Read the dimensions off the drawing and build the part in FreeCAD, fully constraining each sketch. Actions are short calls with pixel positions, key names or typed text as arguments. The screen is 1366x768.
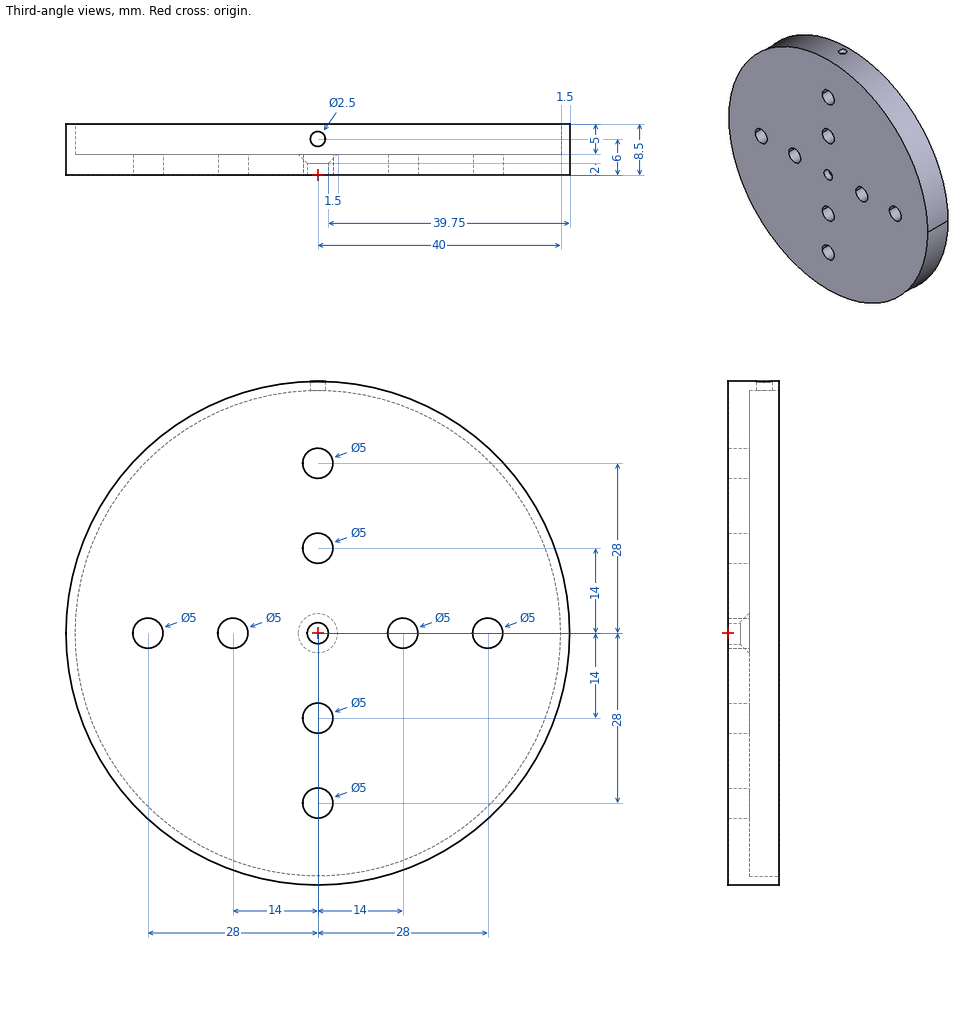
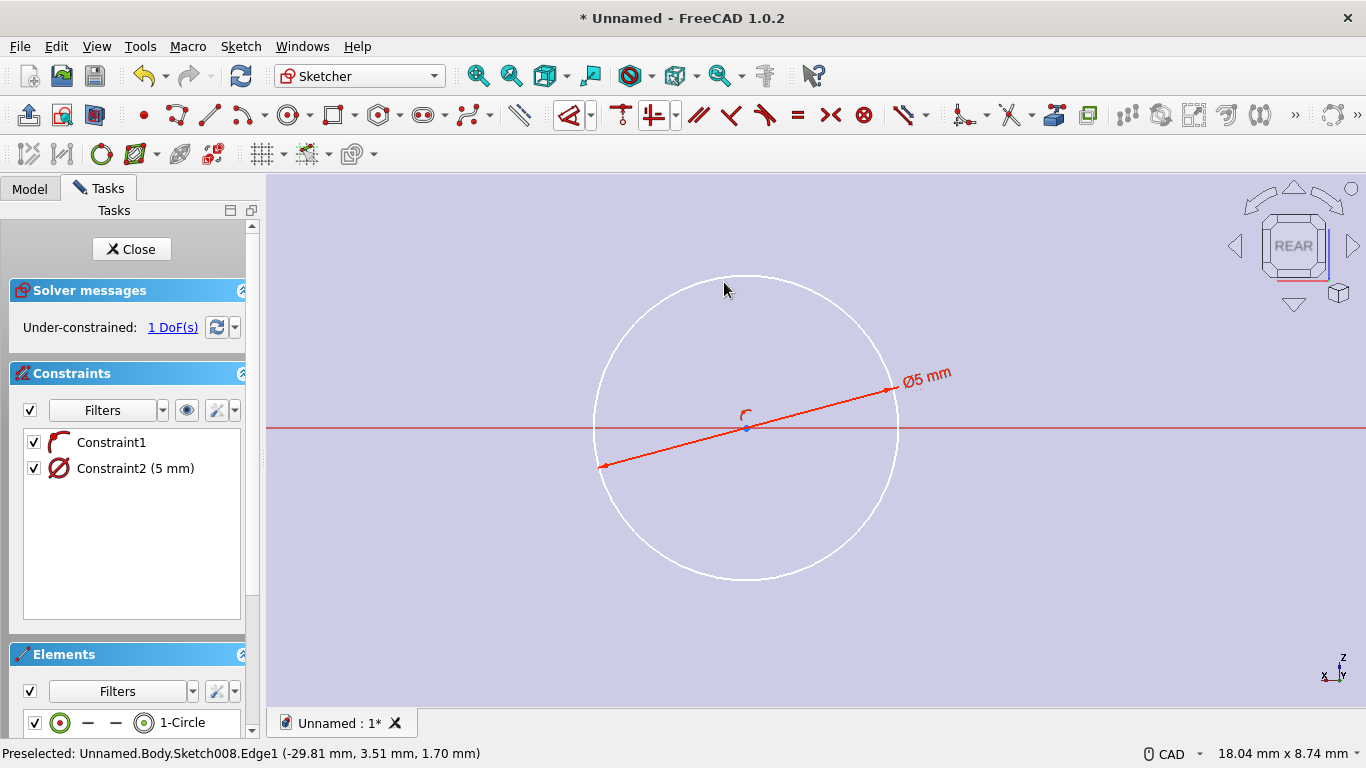
click(746, 428)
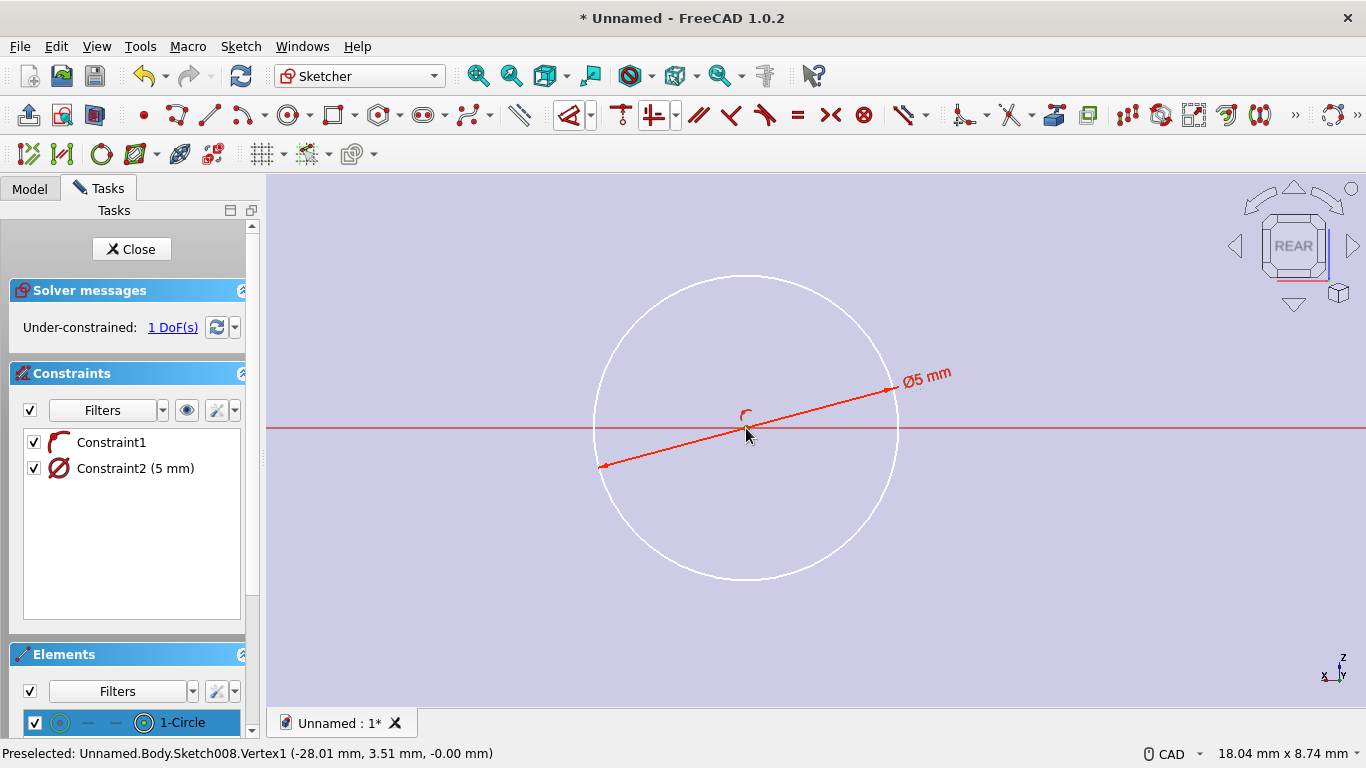
click(590, 116)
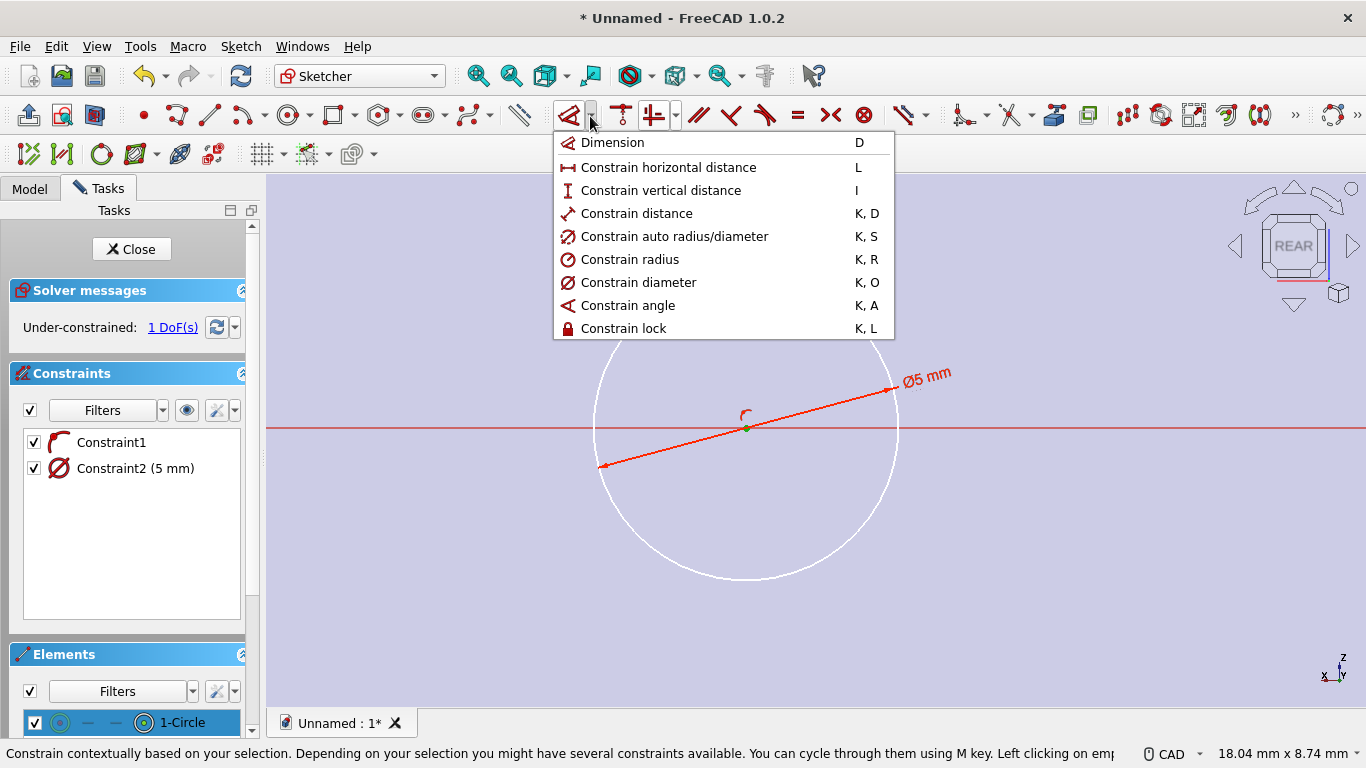
click(724, 168)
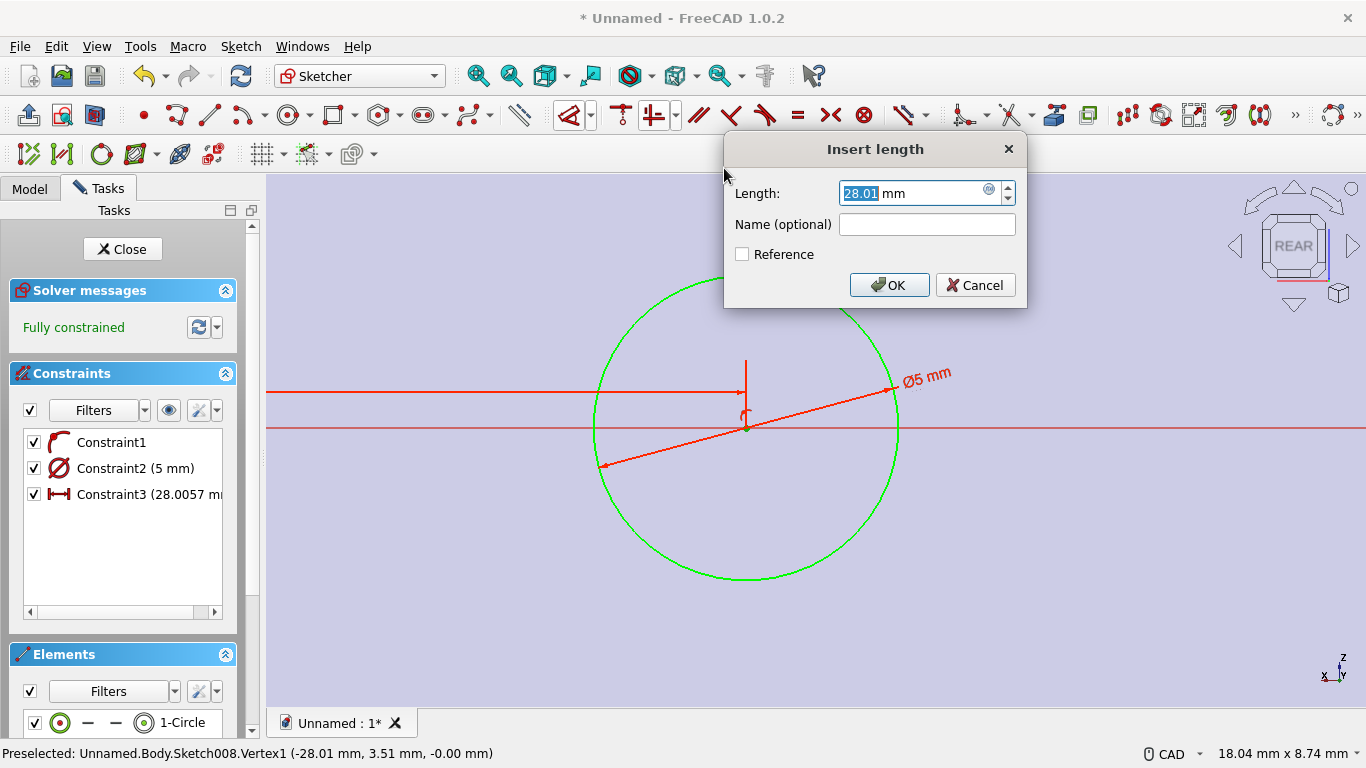
text(28)
key(Return)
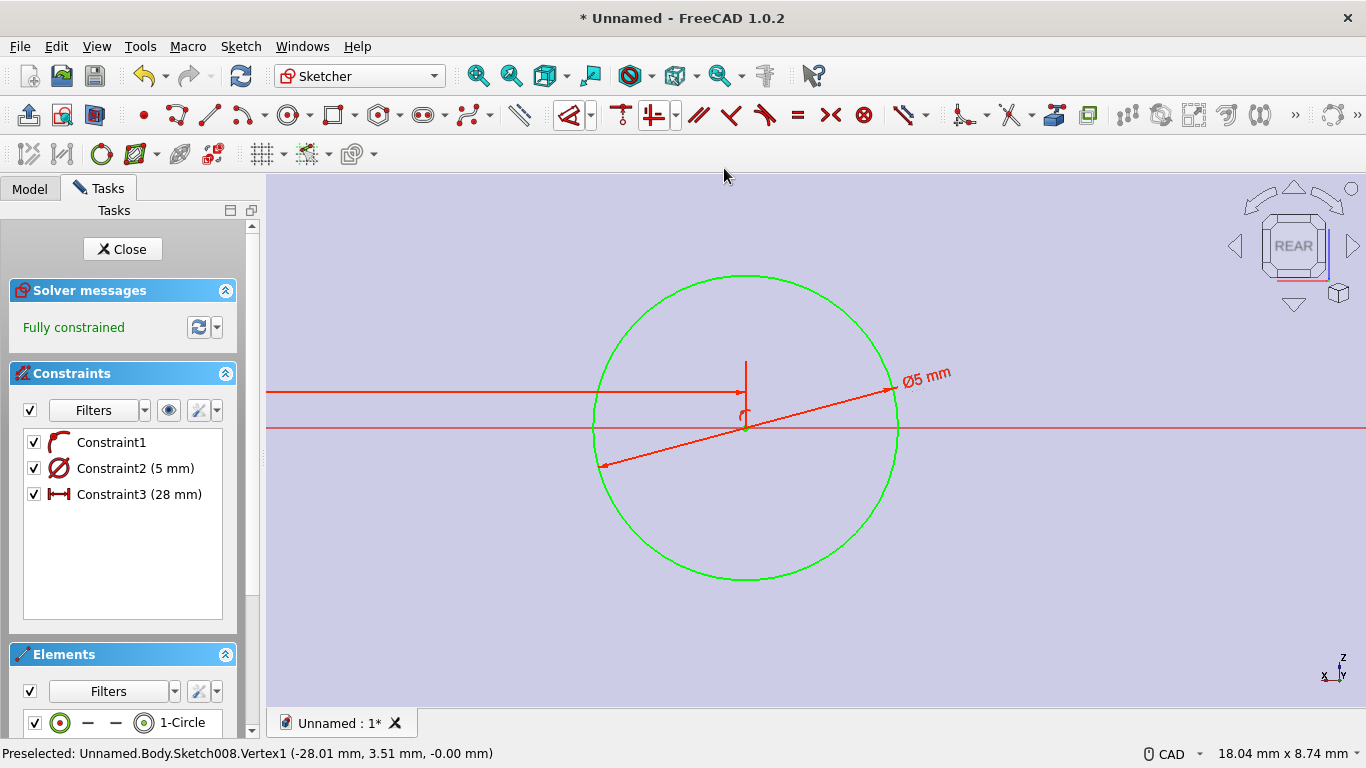
click(123, 249)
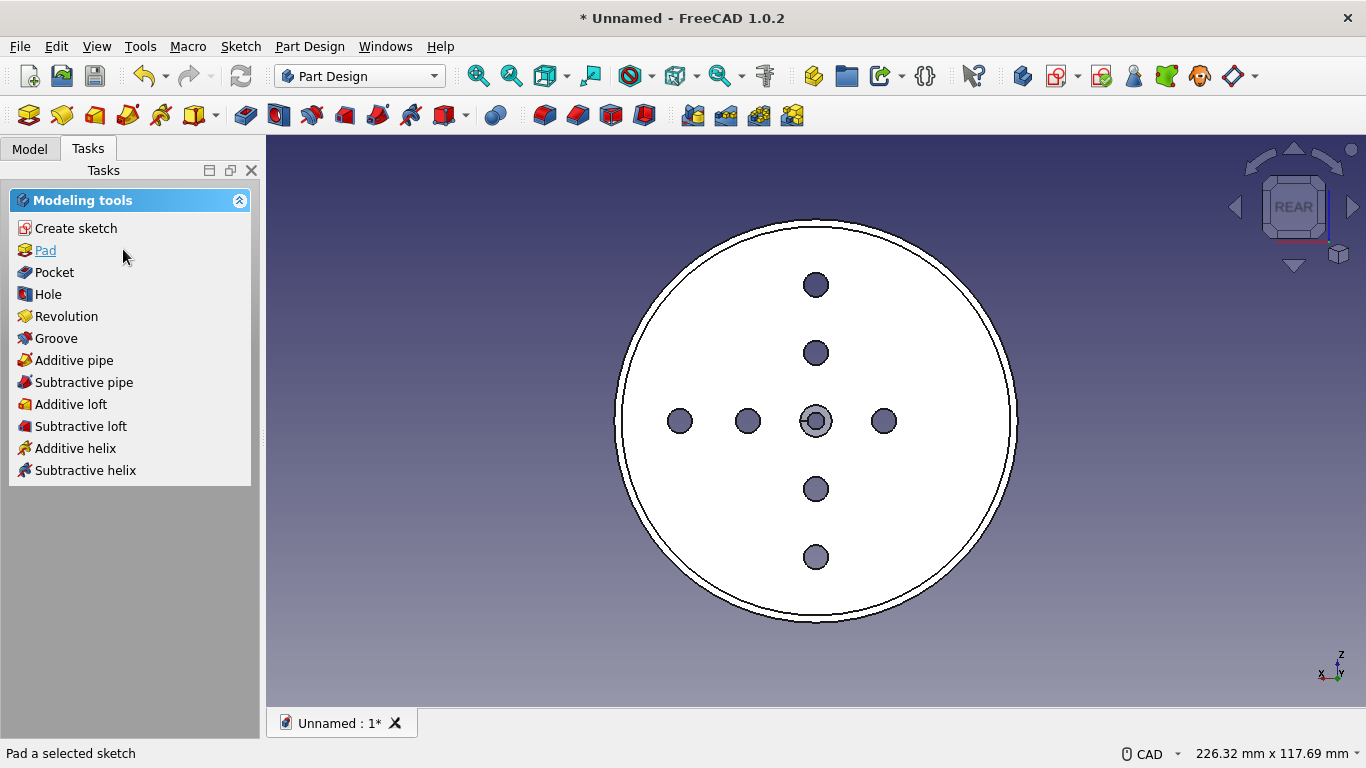
click(246, 116)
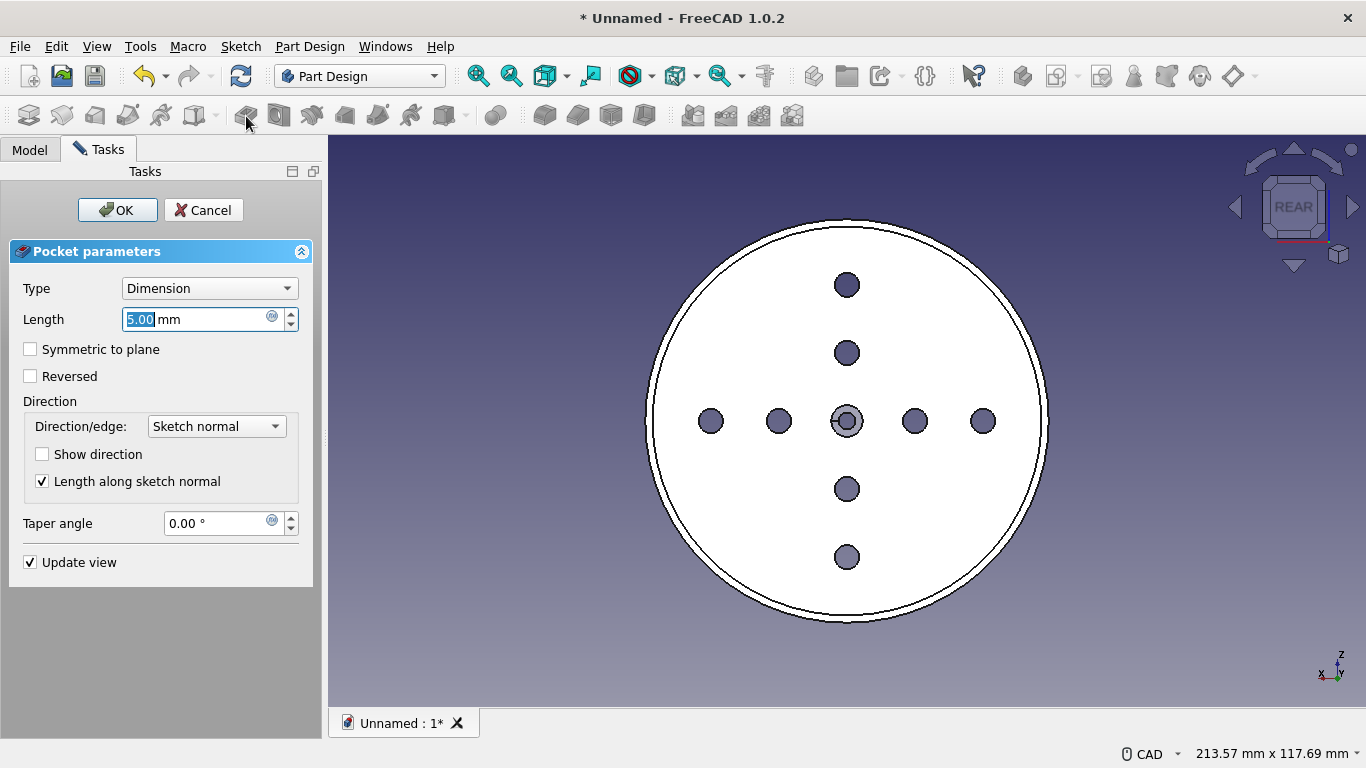
click(210, 288)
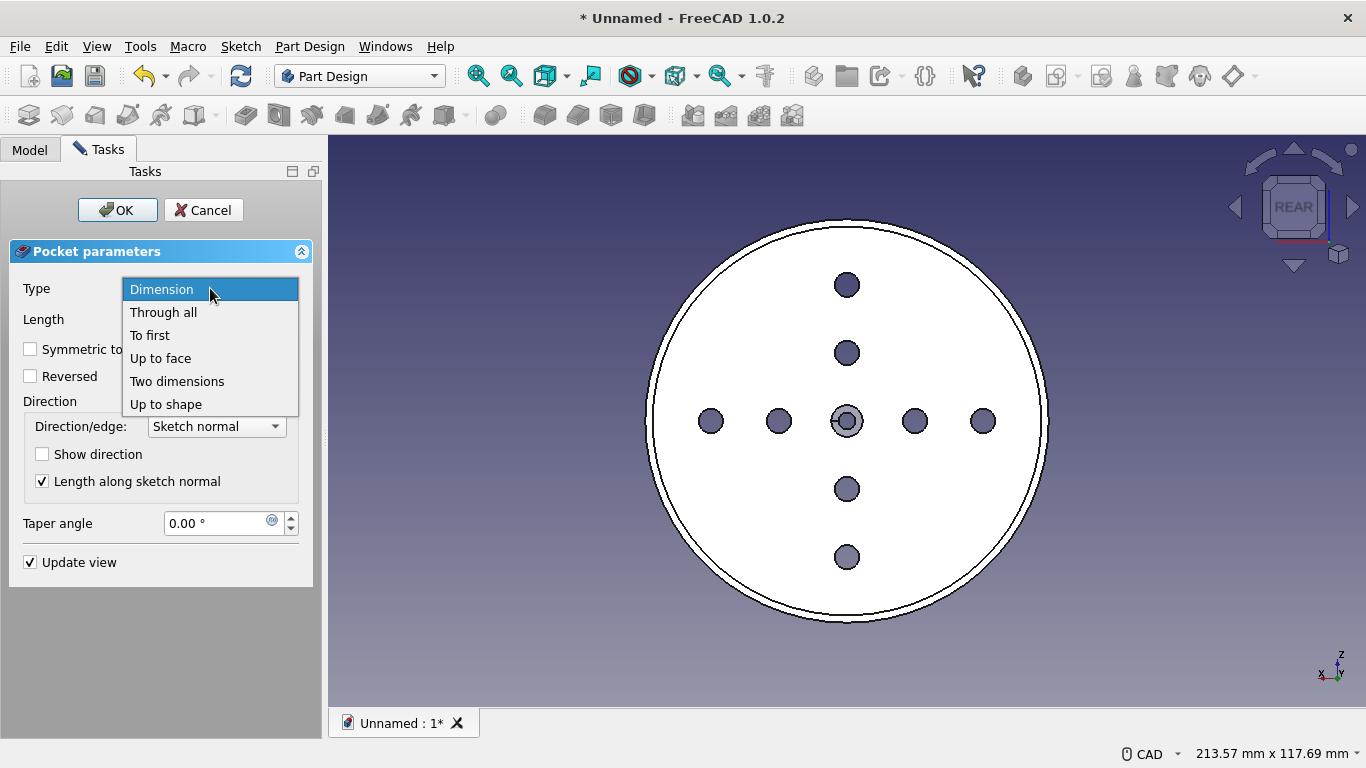
click(208, 336)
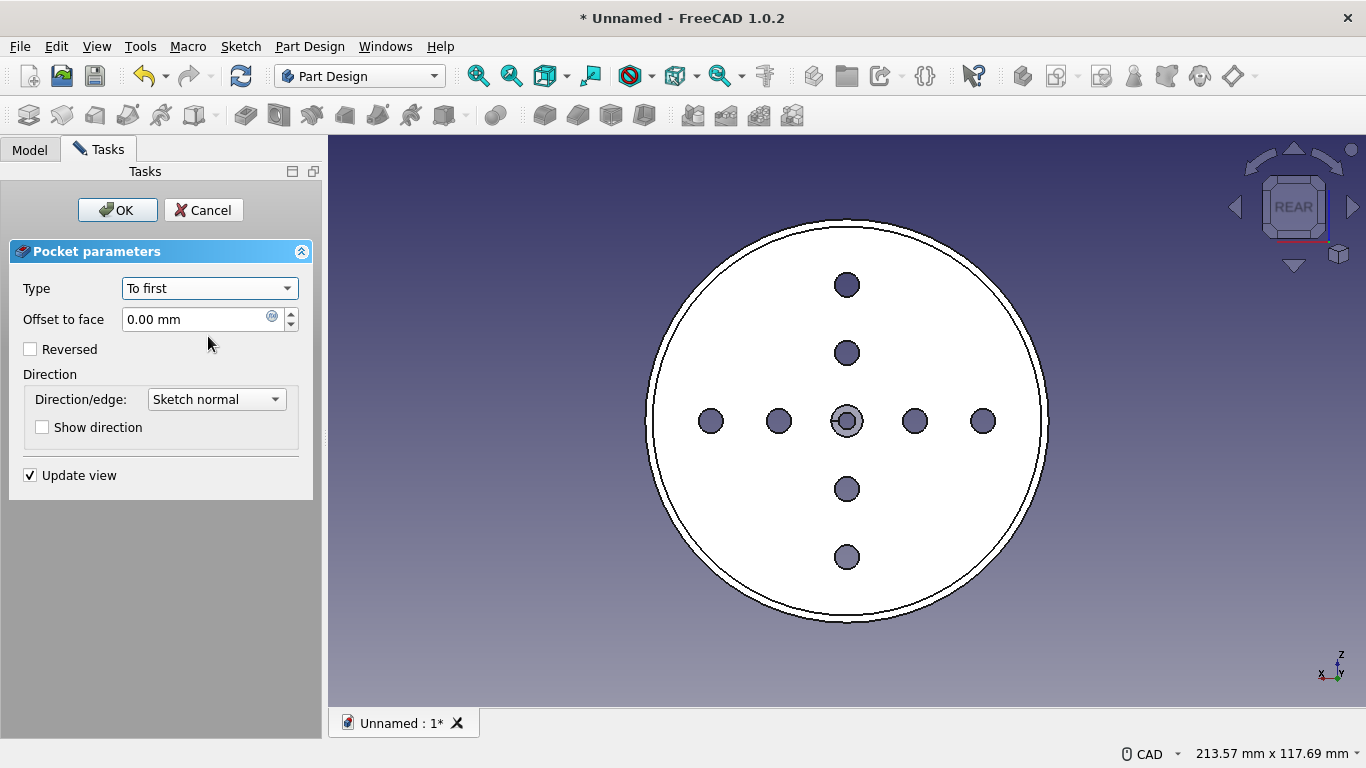
click(118, 210)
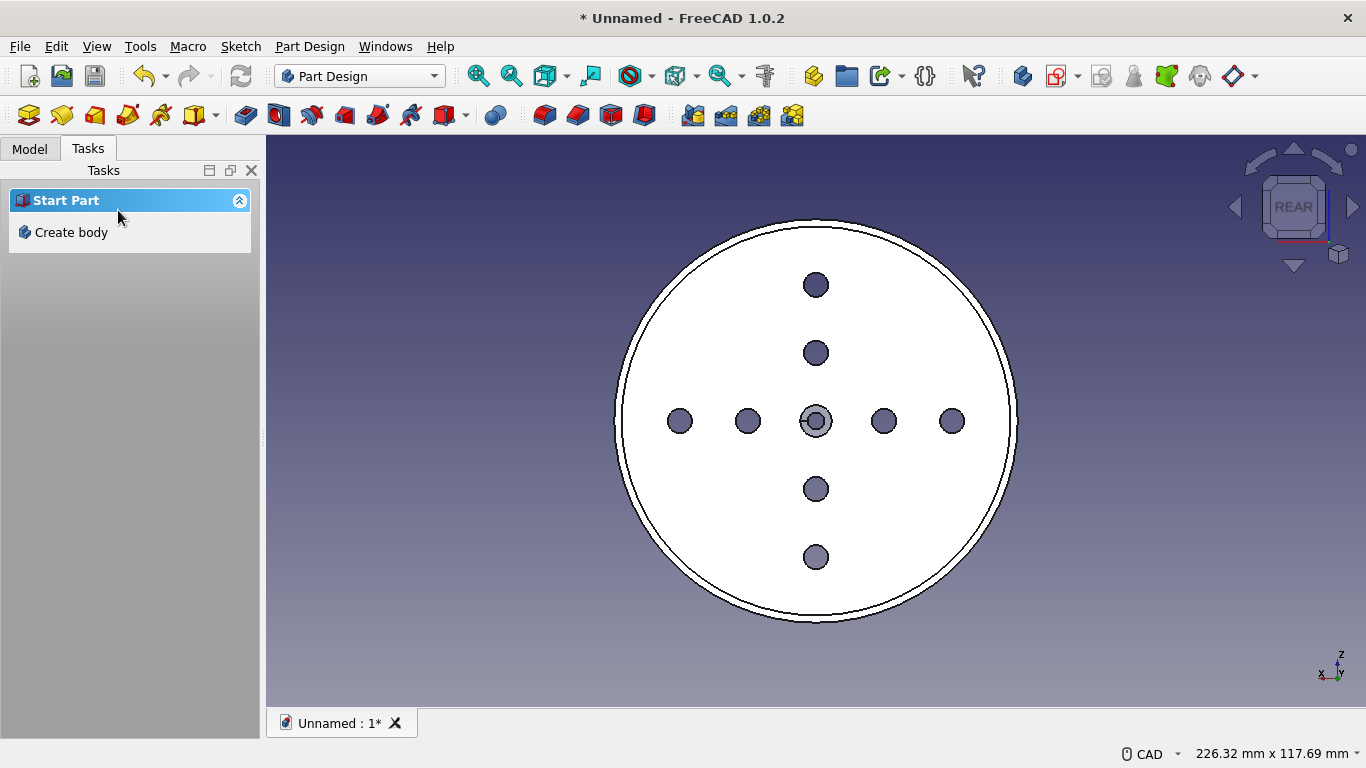
click(30, 148)